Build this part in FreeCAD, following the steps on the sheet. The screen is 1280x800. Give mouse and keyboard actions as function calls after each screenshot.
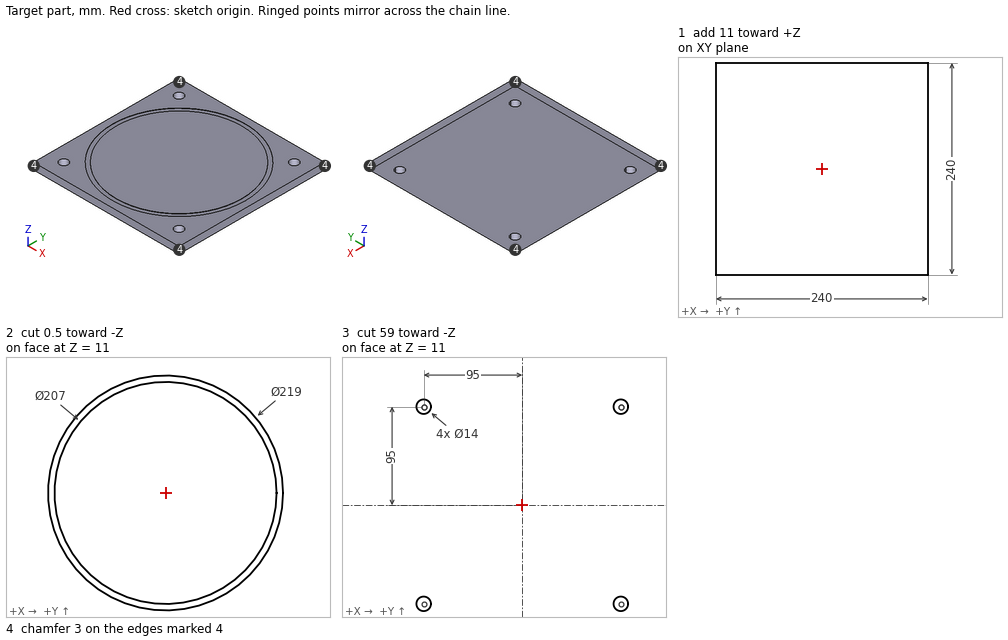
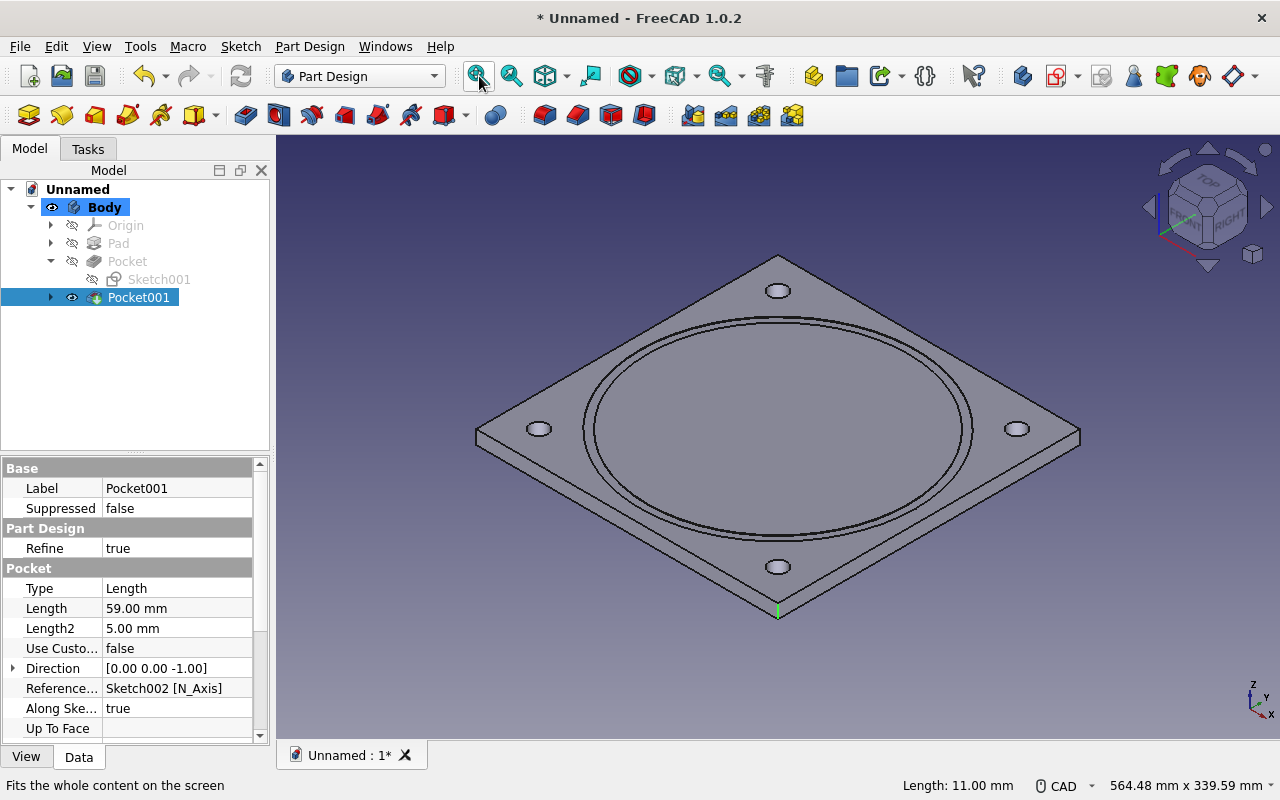
scroll(778, 262, up, 4)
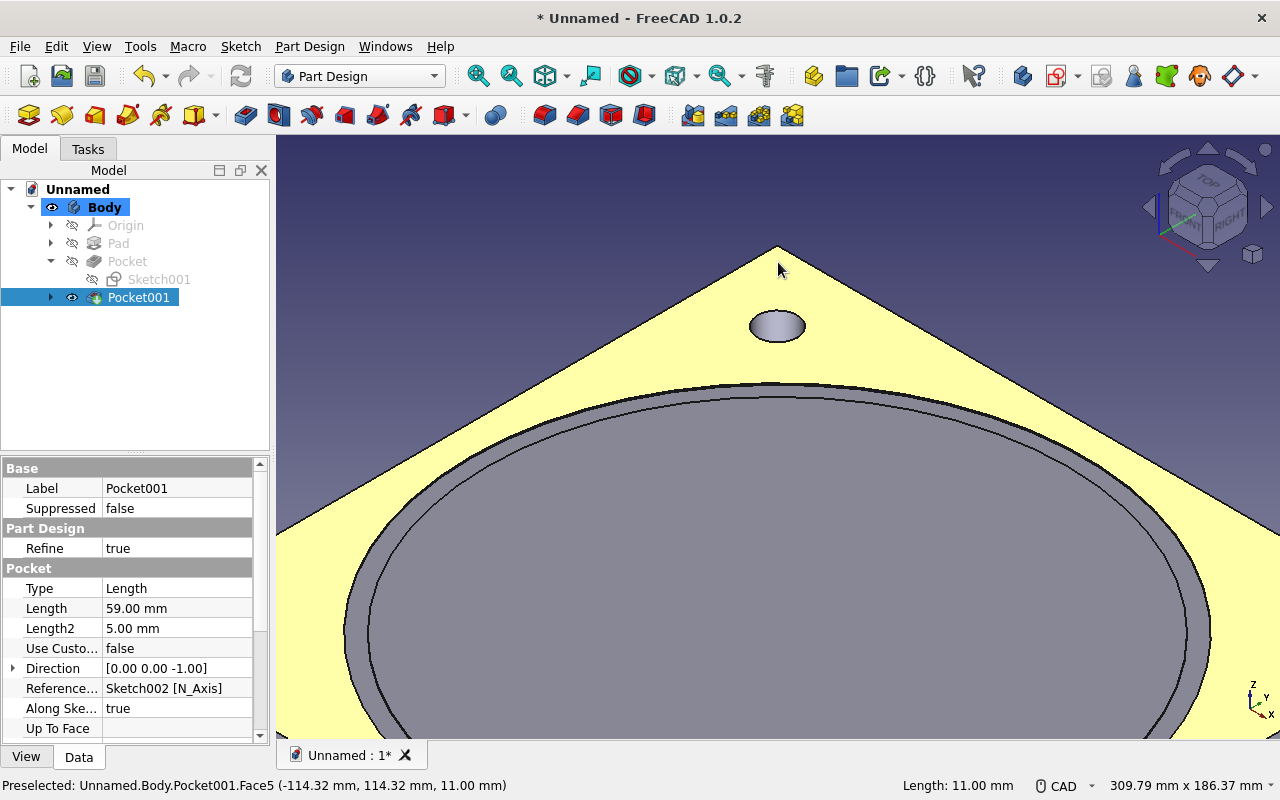
click(479, 76)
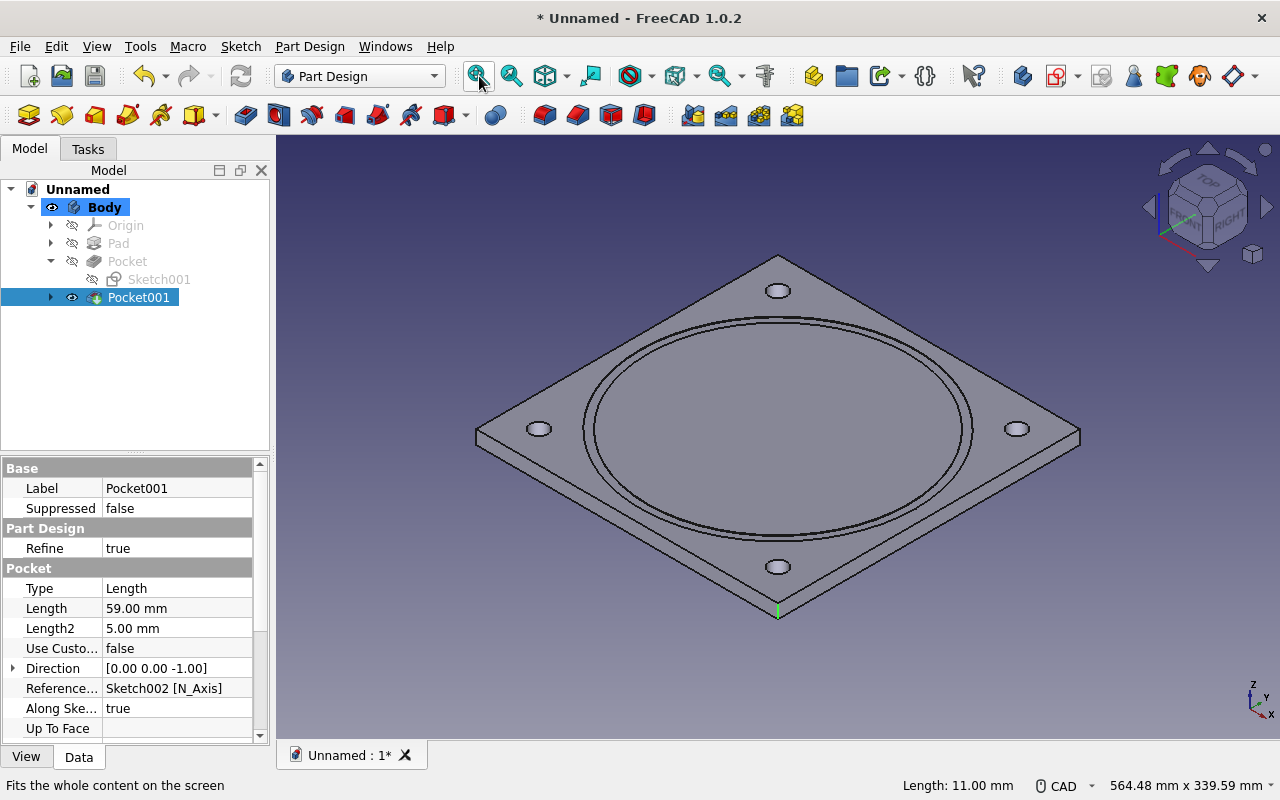
key(2)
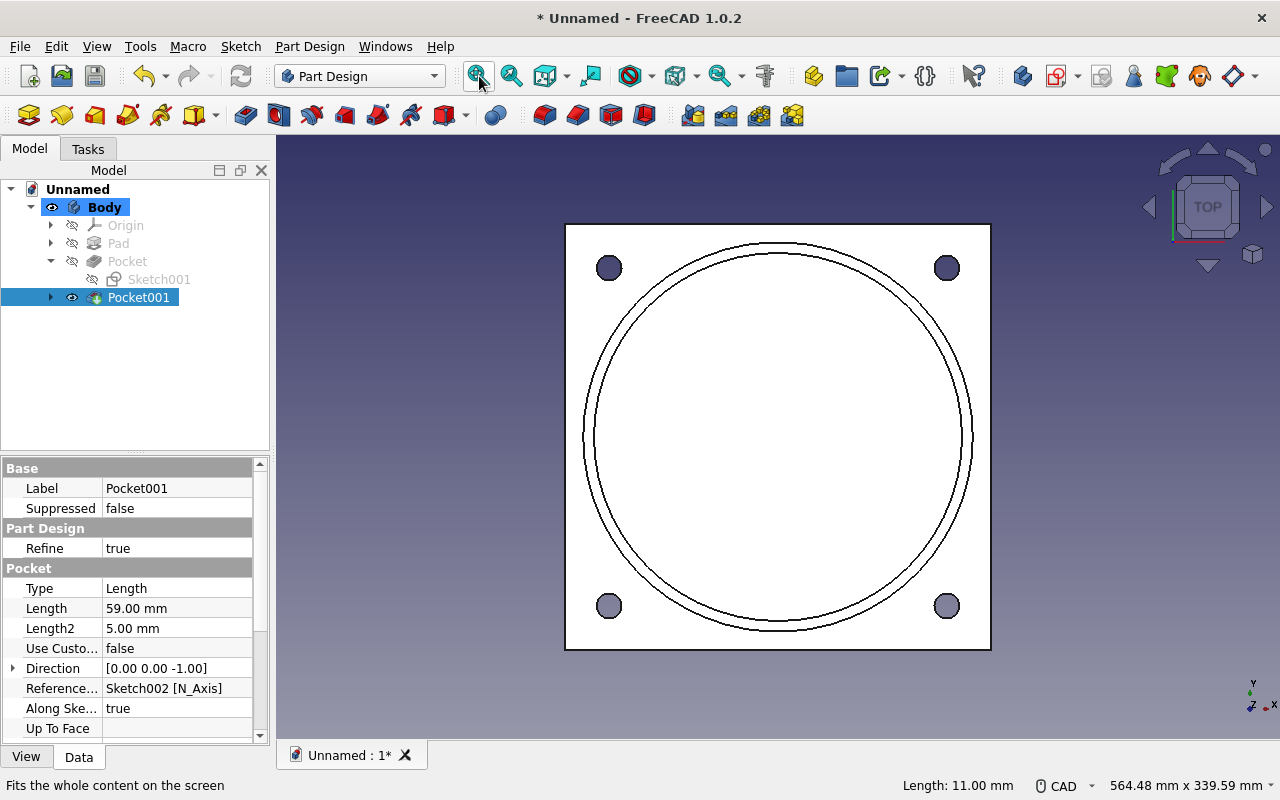
scroll(565, 223, up, 4)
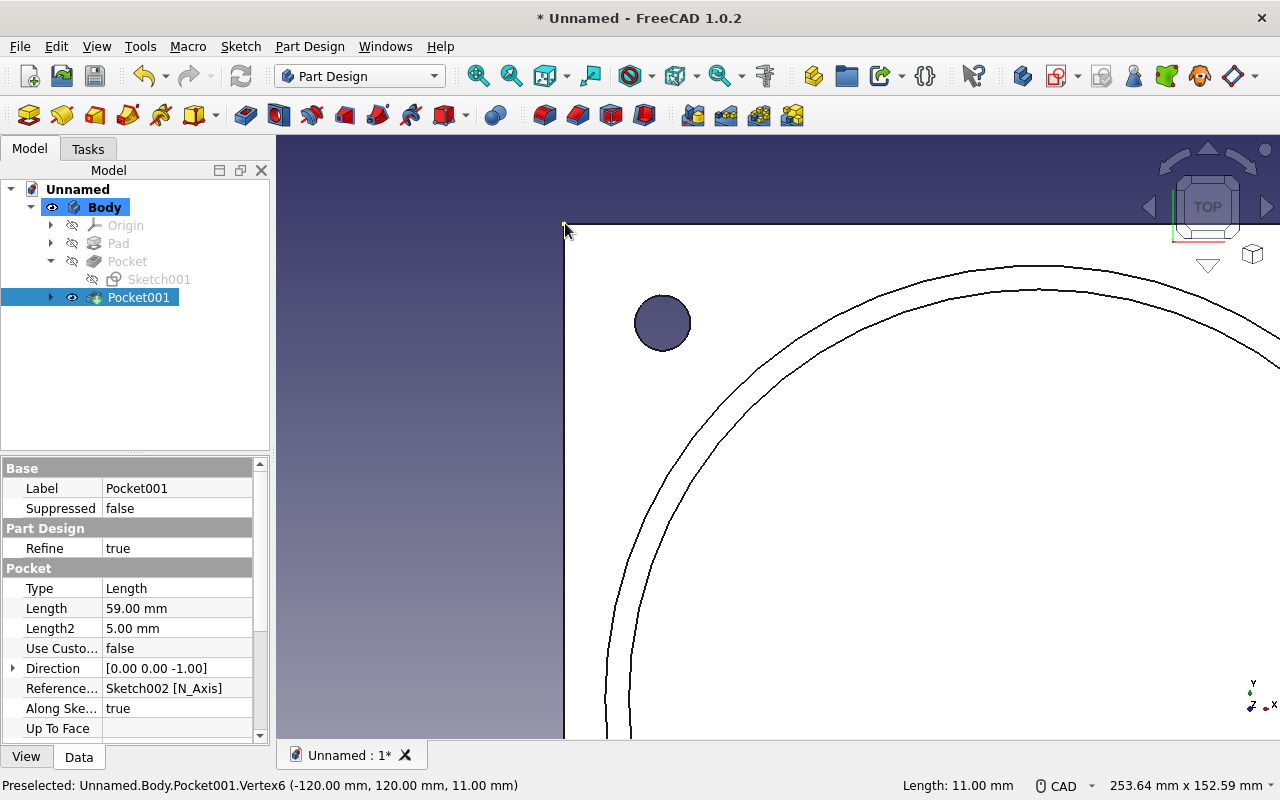
click(479, 76)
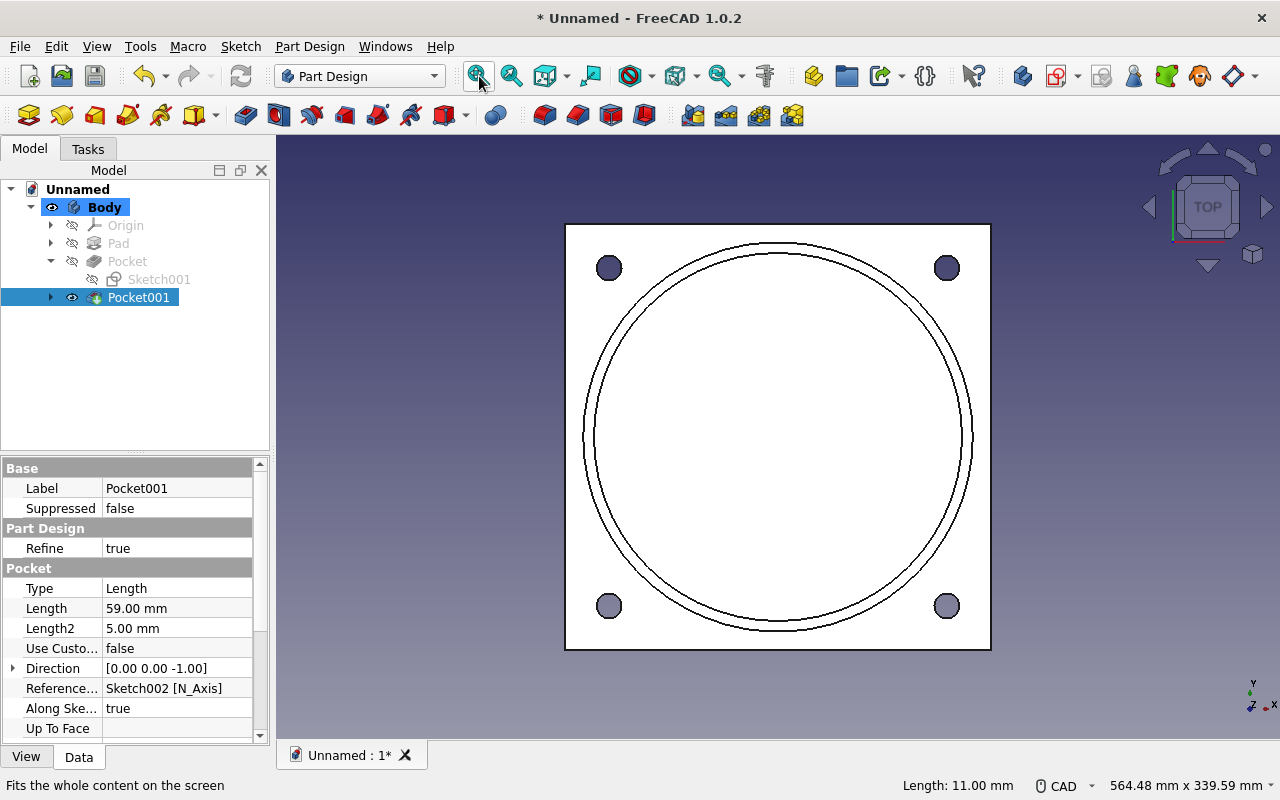
key(1)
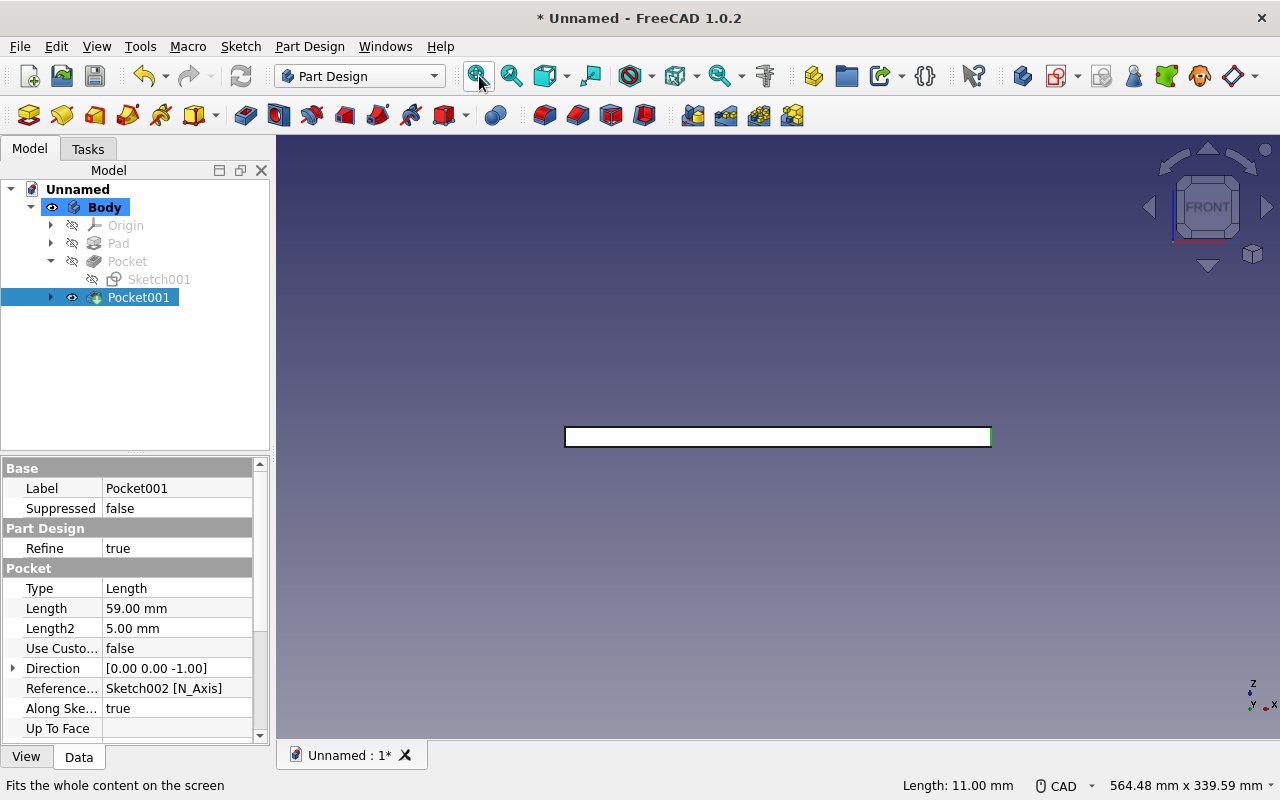
click(479, 76)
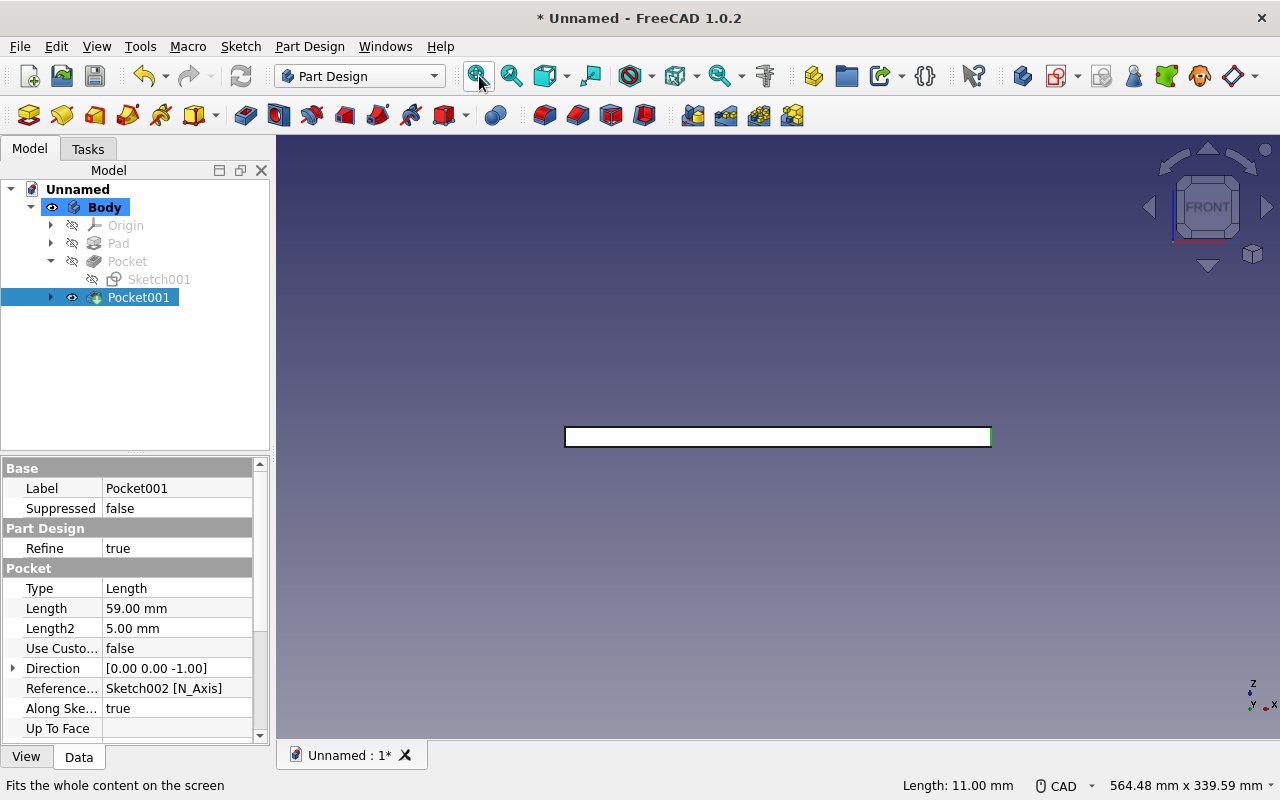
click(565, 436, ctrl)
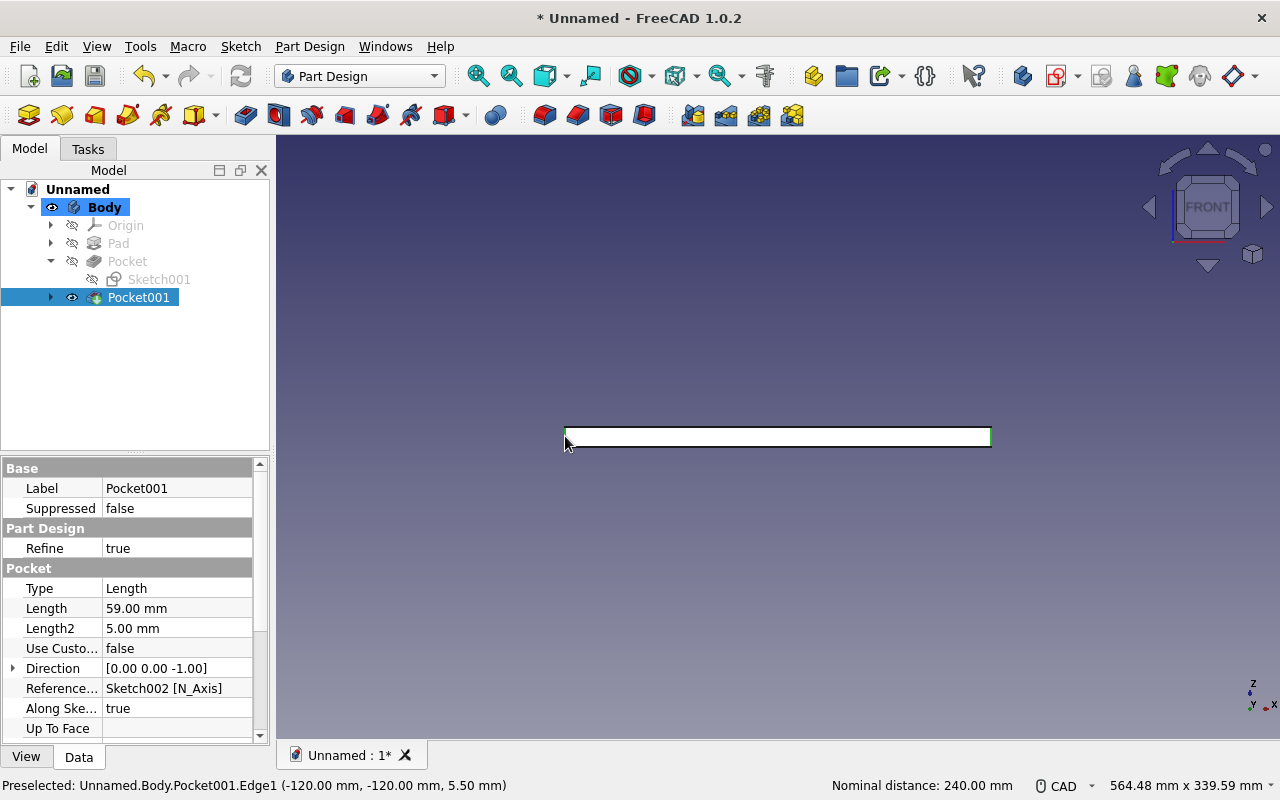
scroll(565, 436, up, 4)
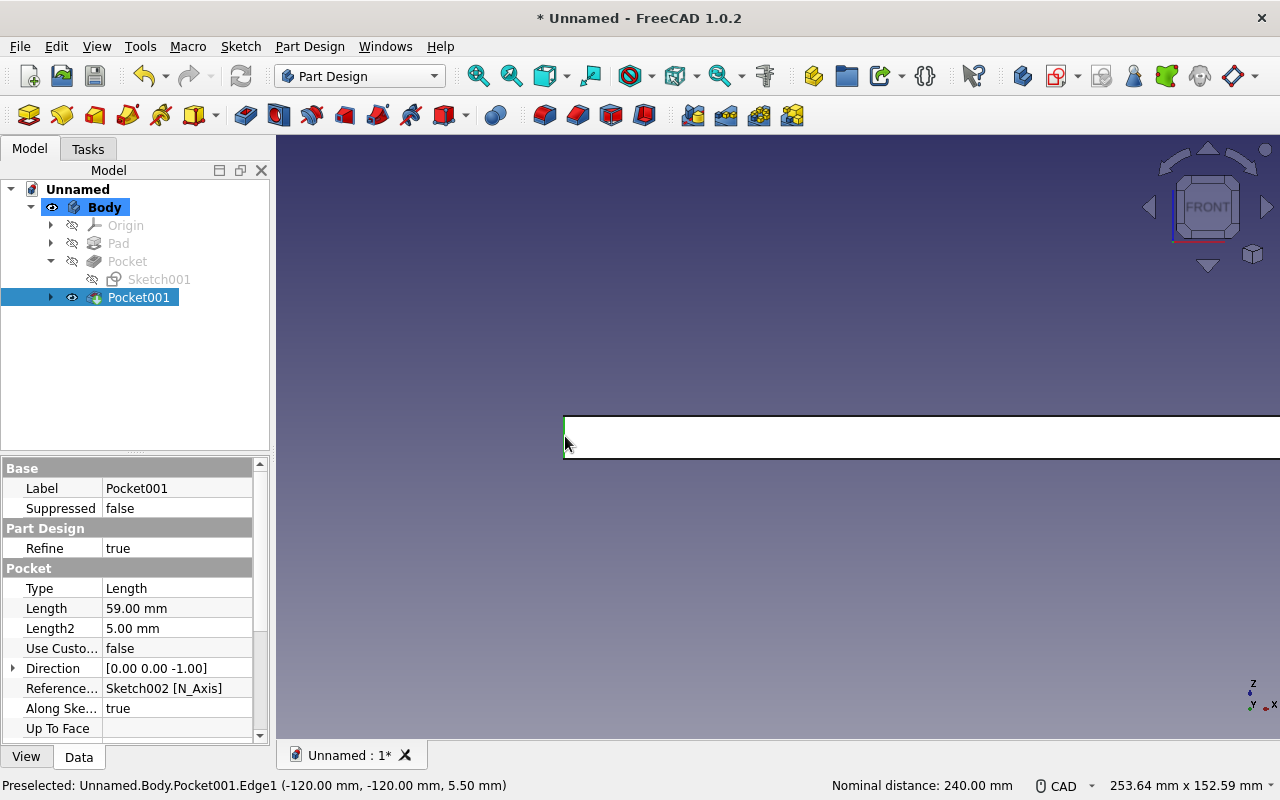
click(479, 76)